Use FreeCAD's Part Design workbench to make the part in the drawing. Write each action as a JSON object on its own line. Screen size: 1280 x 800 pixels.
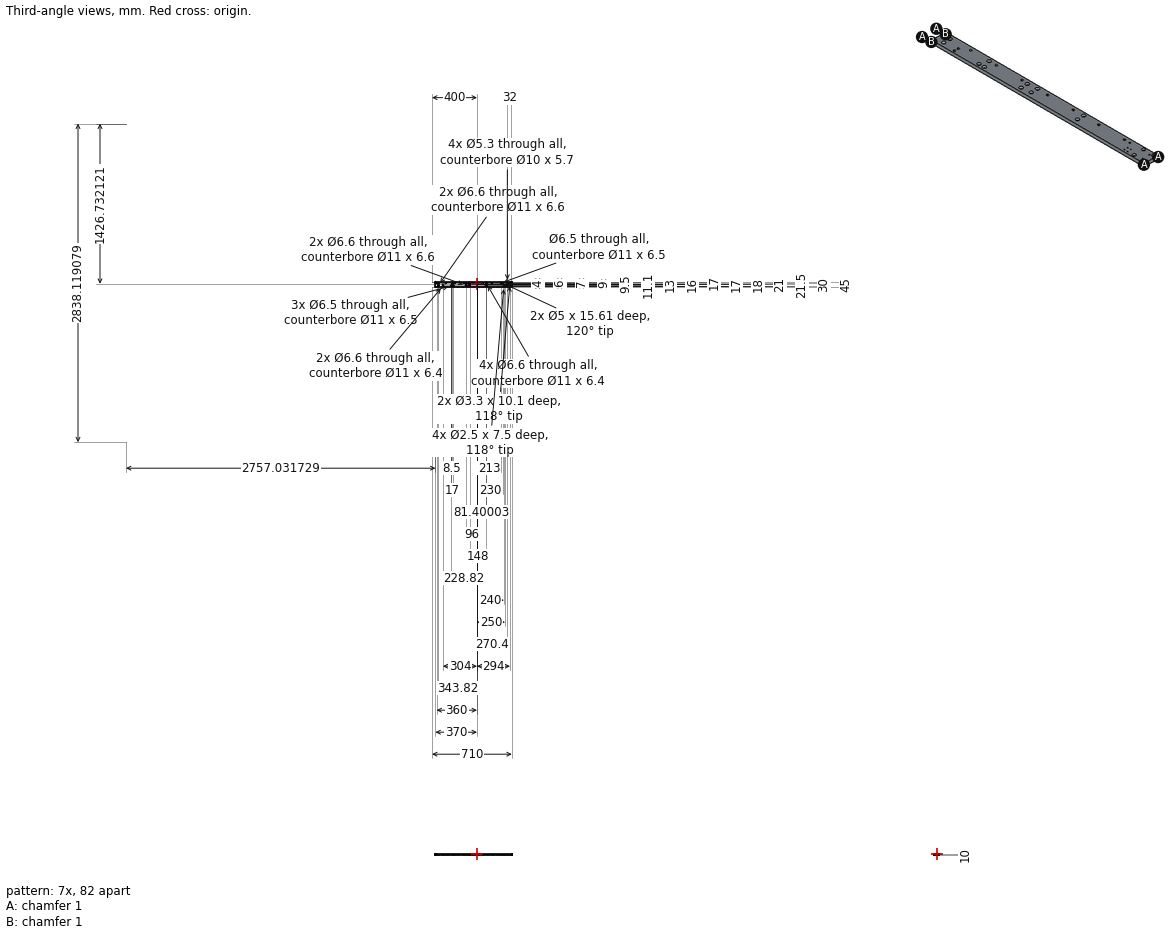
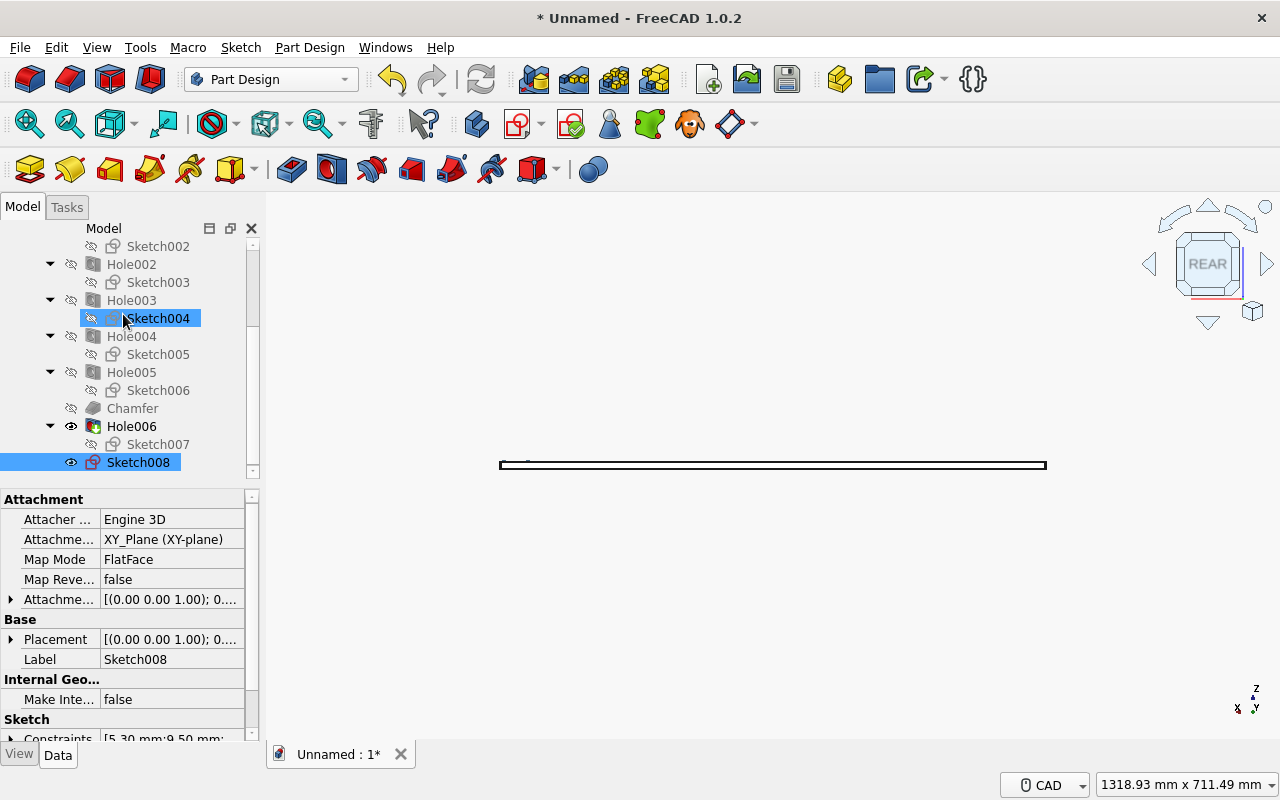
{"action": "left_click", "coordinate": [332, 170]}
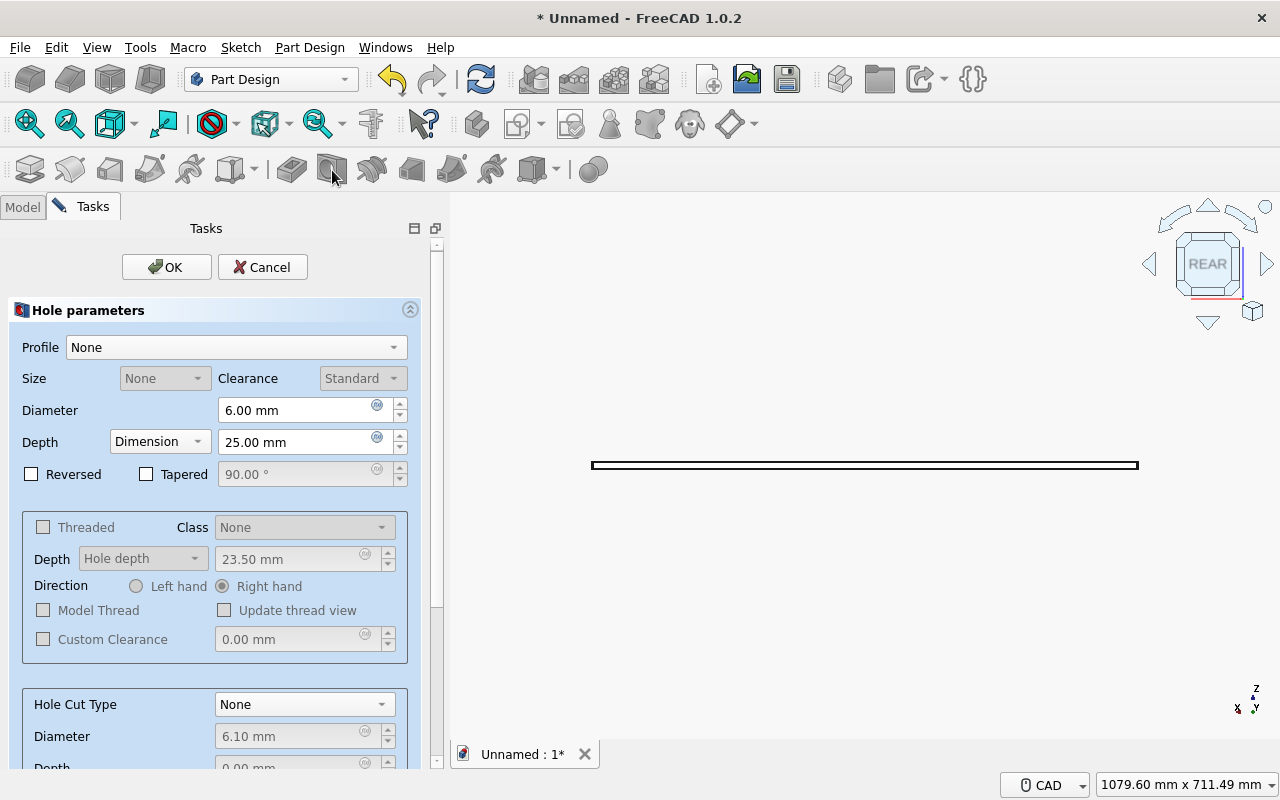
{"action": "triple_click", "coordinate": [305, 410]}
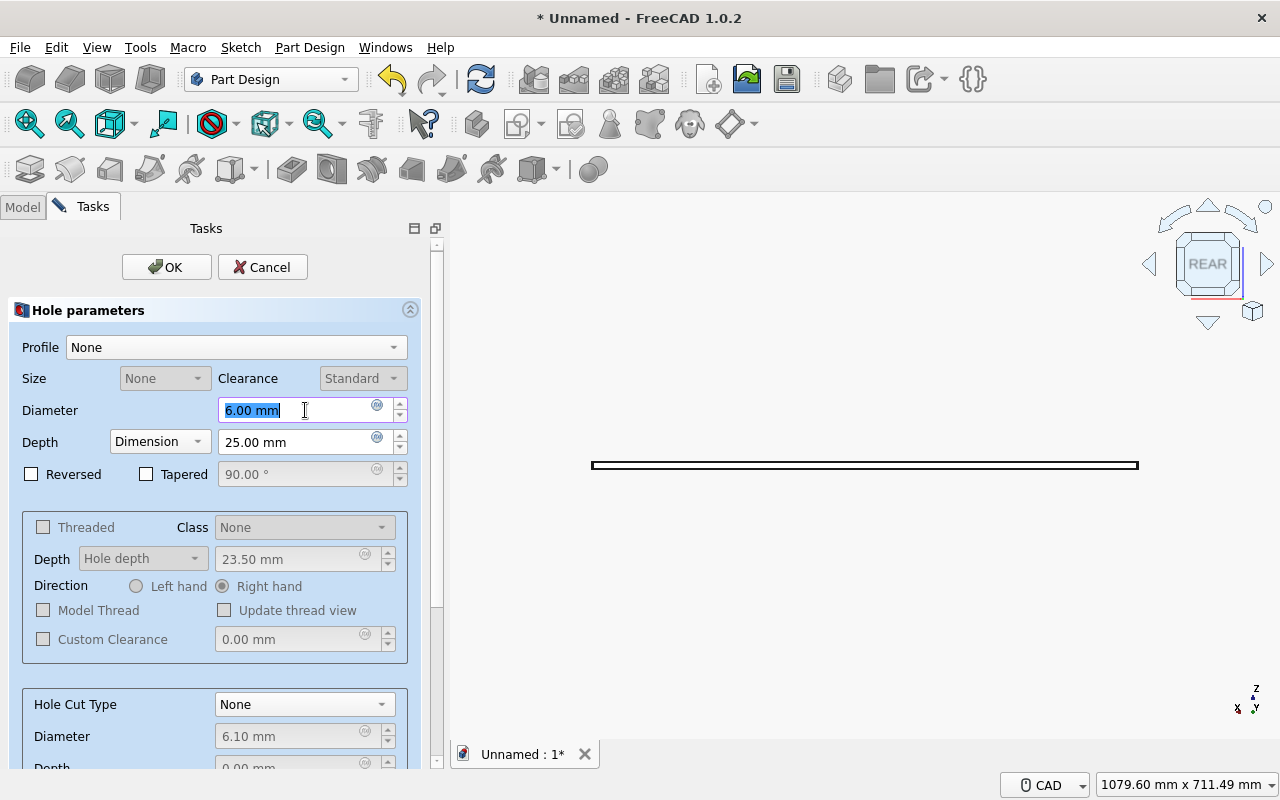
{"action": "type", "text": "5.3"}
{"action": "key", "text": "Tab"}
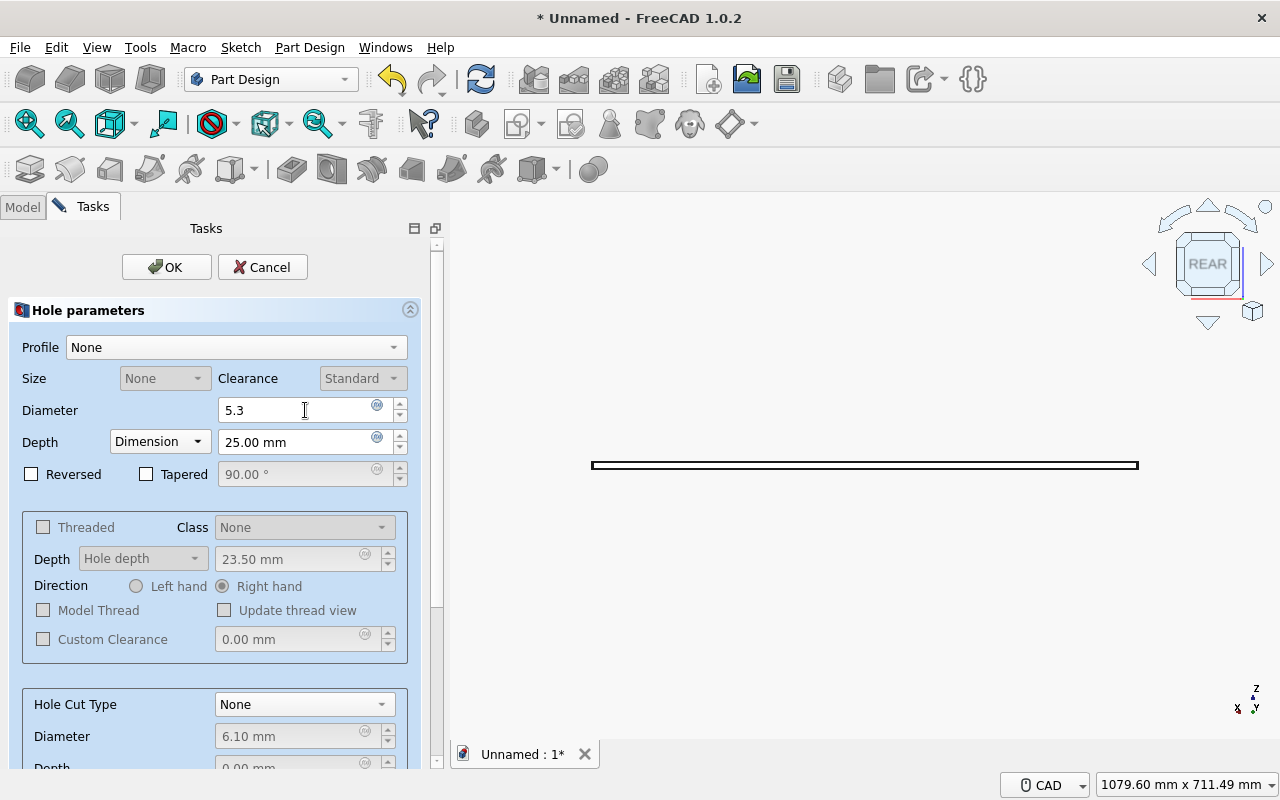
{"action": "left_click", "coordinate": [161, 442]}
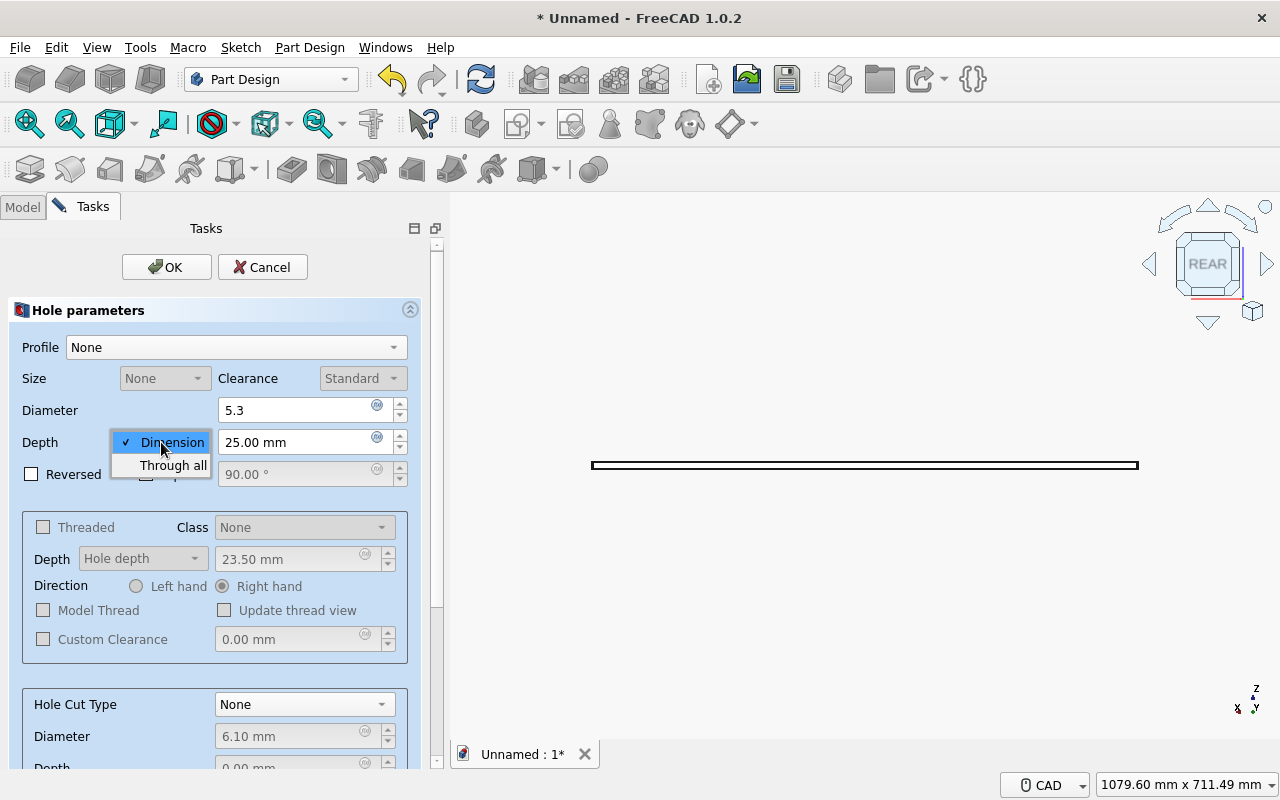
{"action": "left_click", "coordinate": [160, 466]}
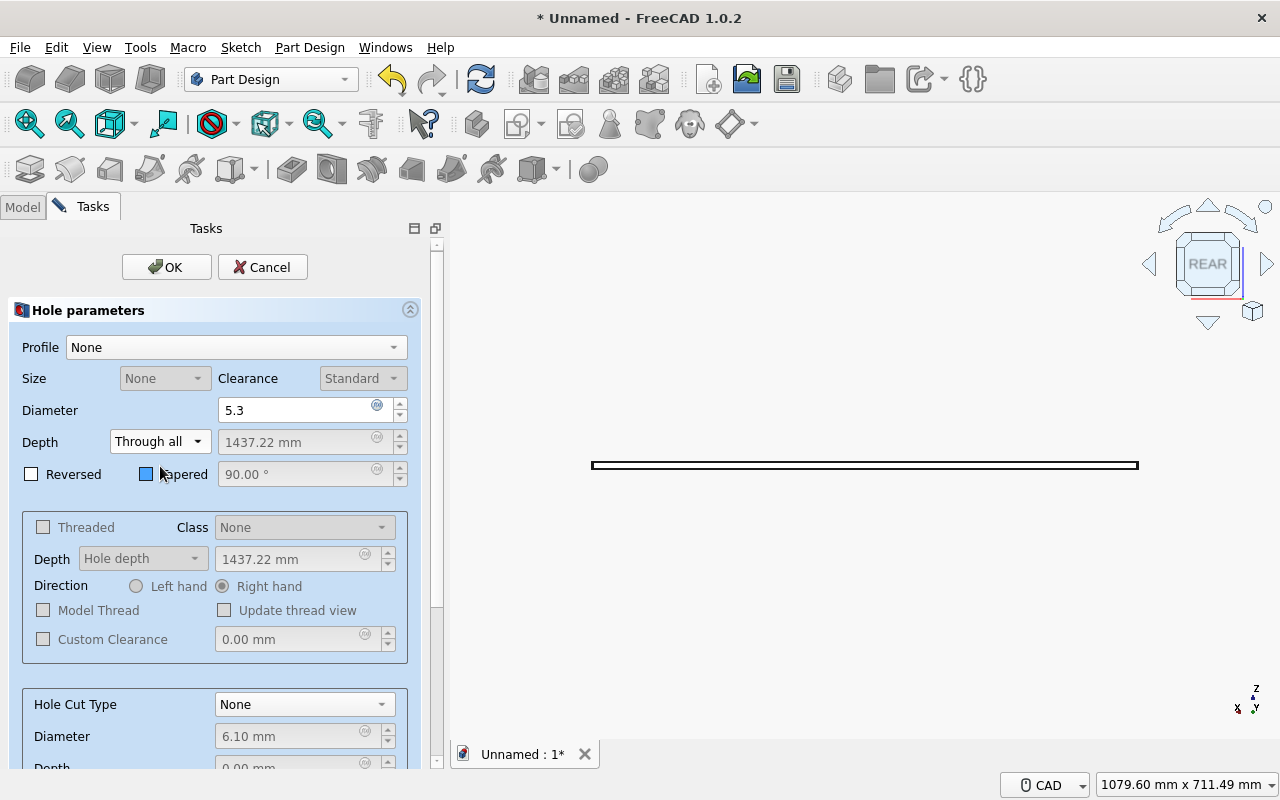
{"action": "left_click", "coordinate": [306, 704]}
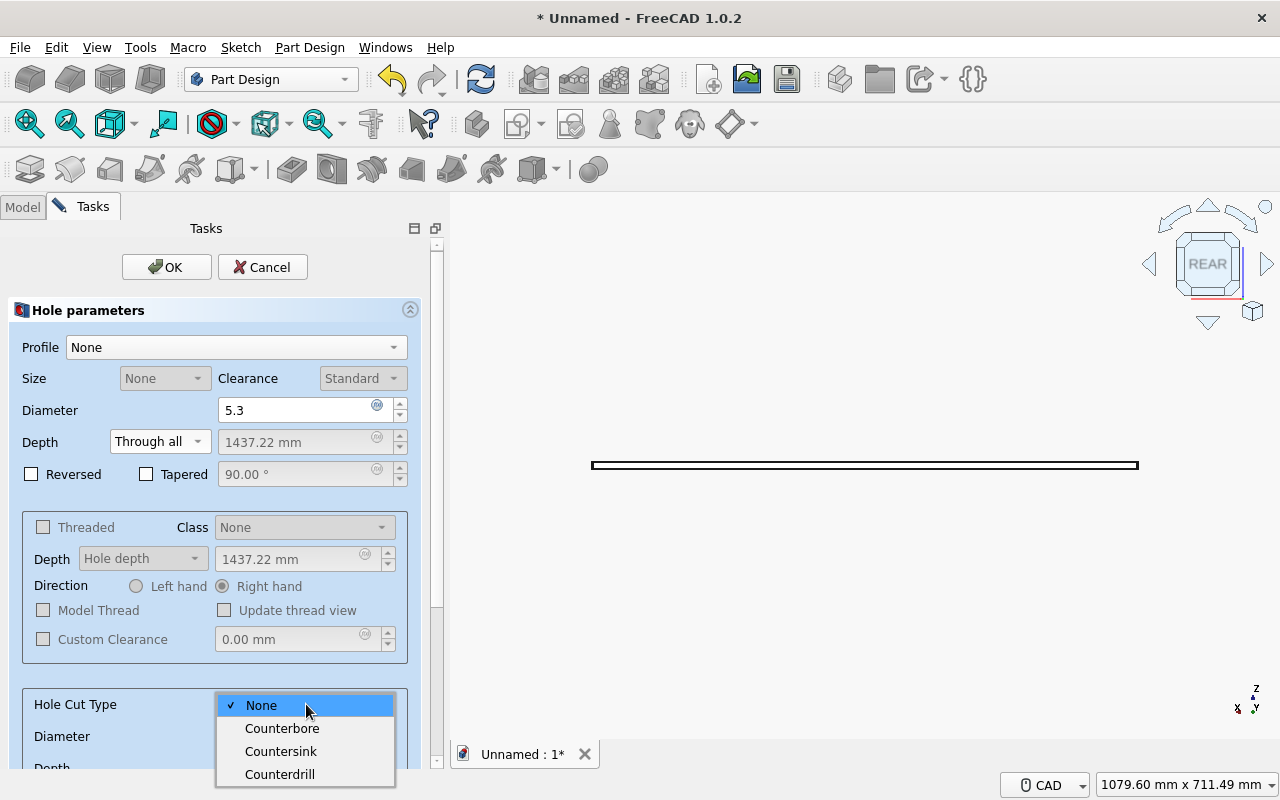
{"action": "left_click", "coordinate": [304, 728]}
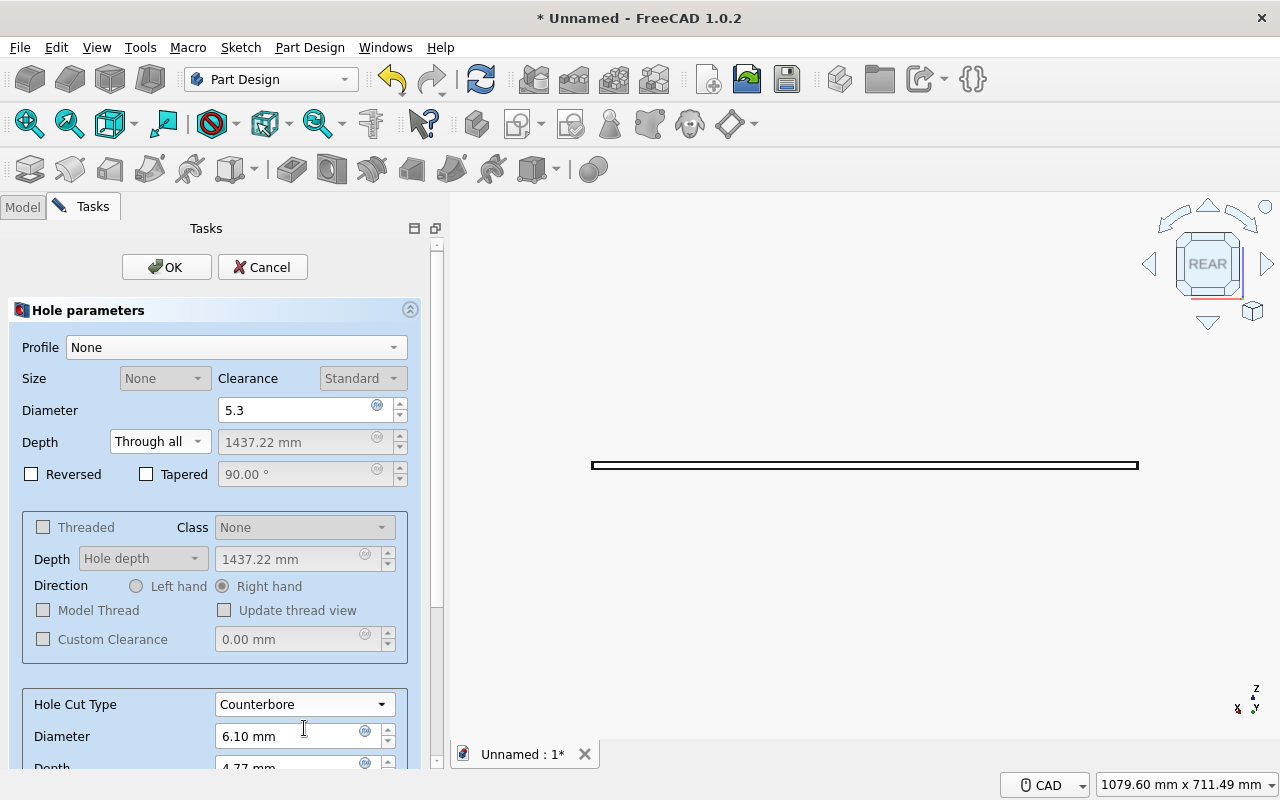
{"action": "triple_click", "coordinate": [298, 736]}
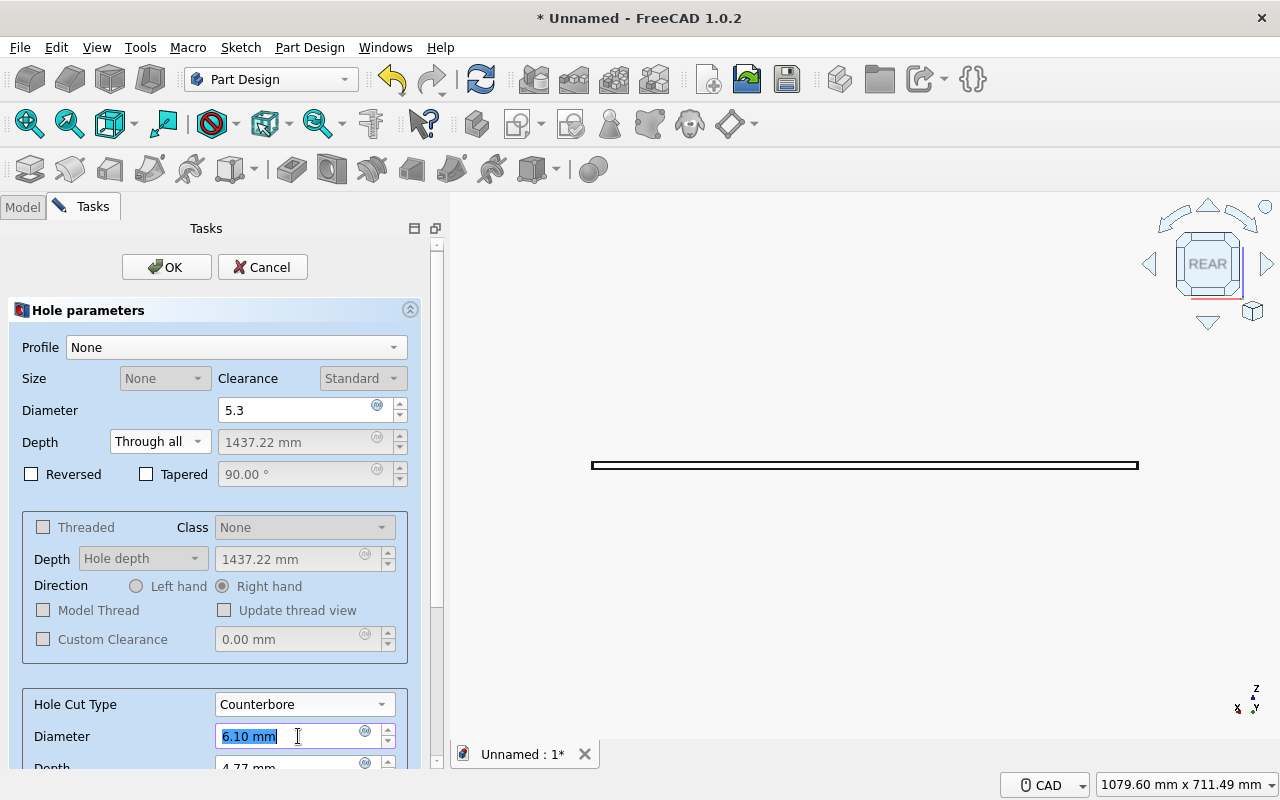
{"action": "type", "text": "10"}
{"action": "key", "text": "Tab"}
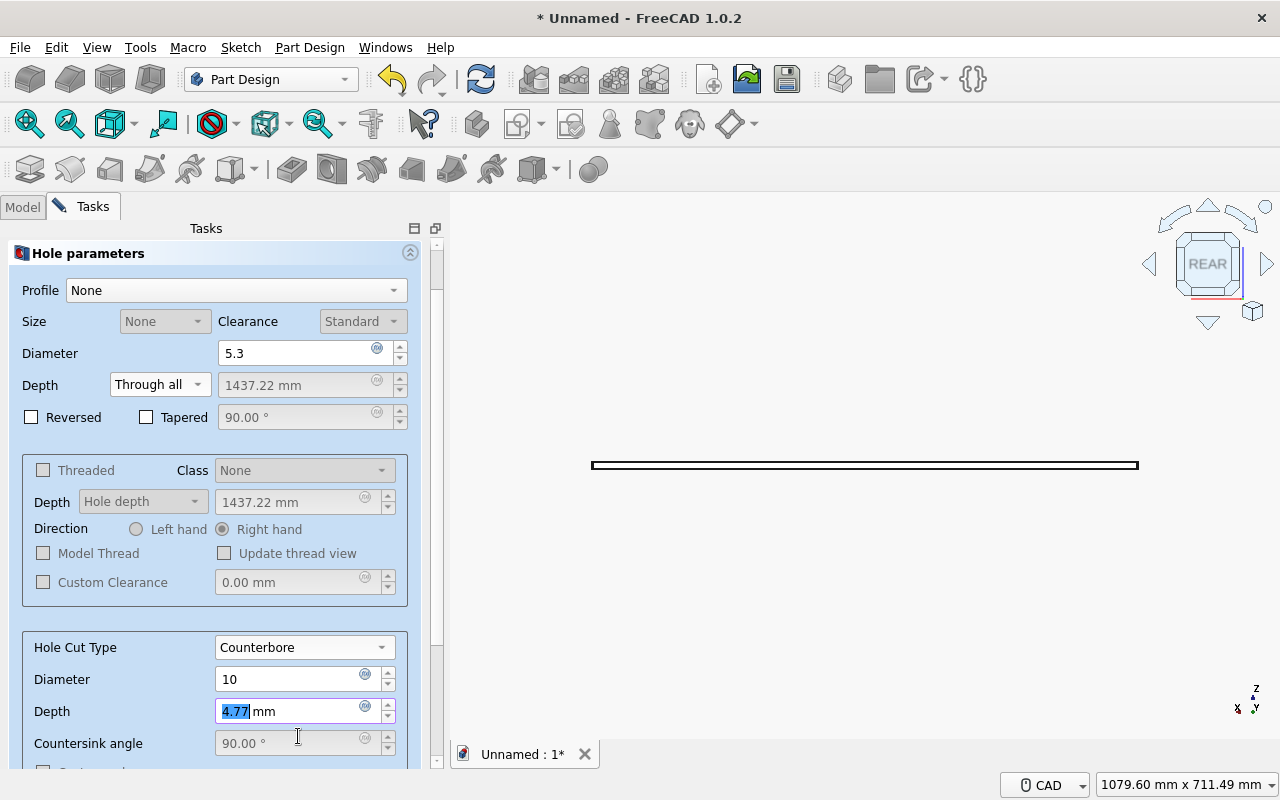
{"action": "type", "text": "5.7"}
{"action": "key", "text": "Tab"}